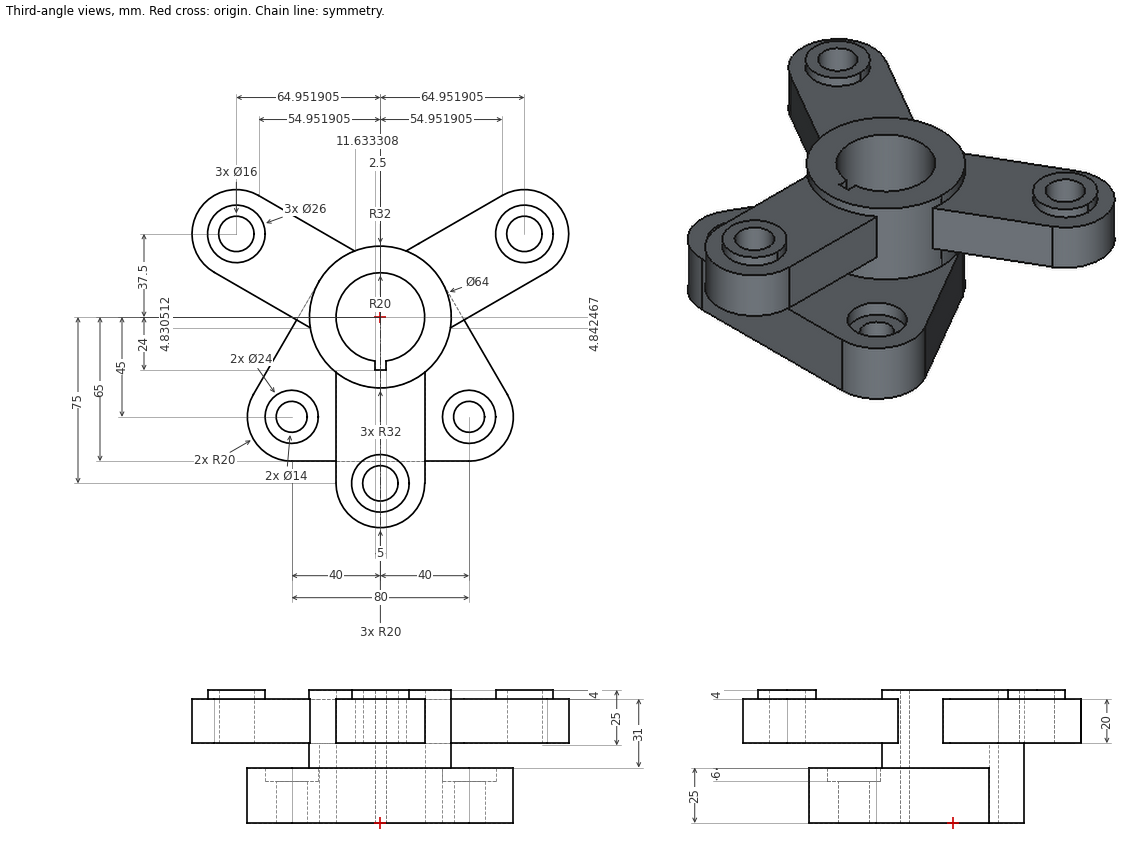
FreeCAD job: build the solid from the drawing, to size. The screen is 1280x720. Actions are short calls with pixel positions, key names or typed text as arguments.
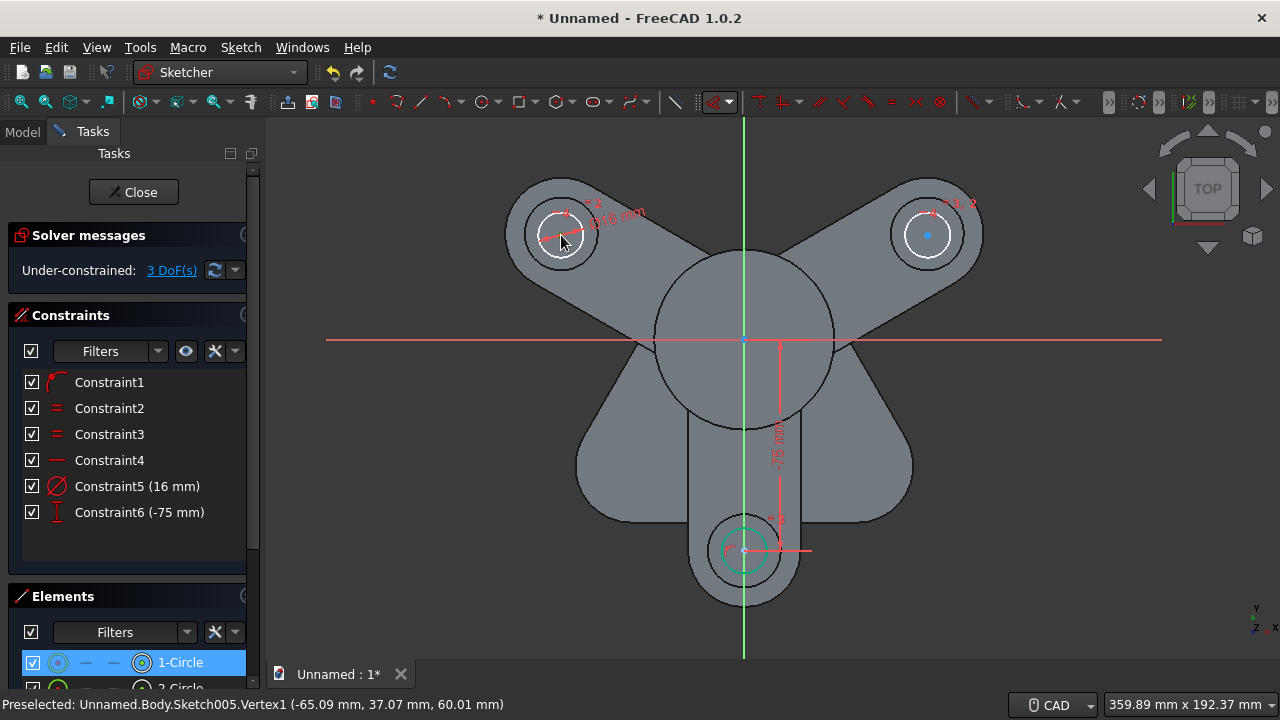
click(732, 102)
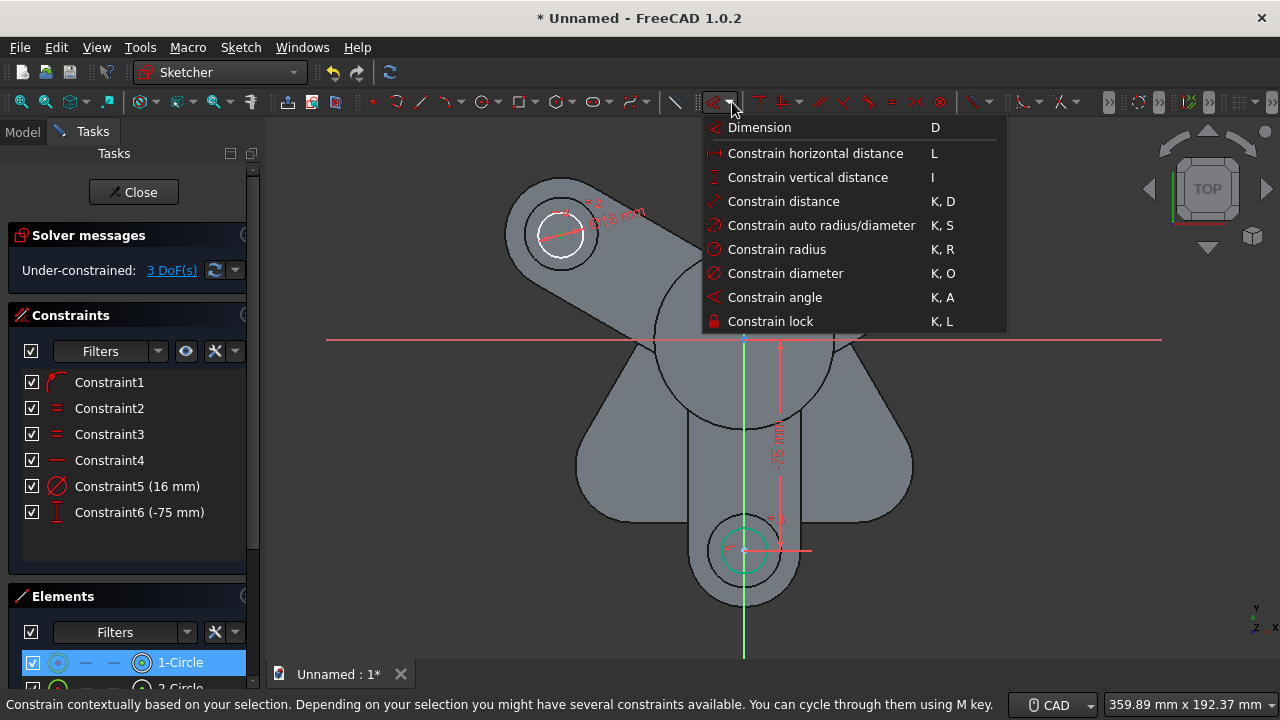
click(855, 177)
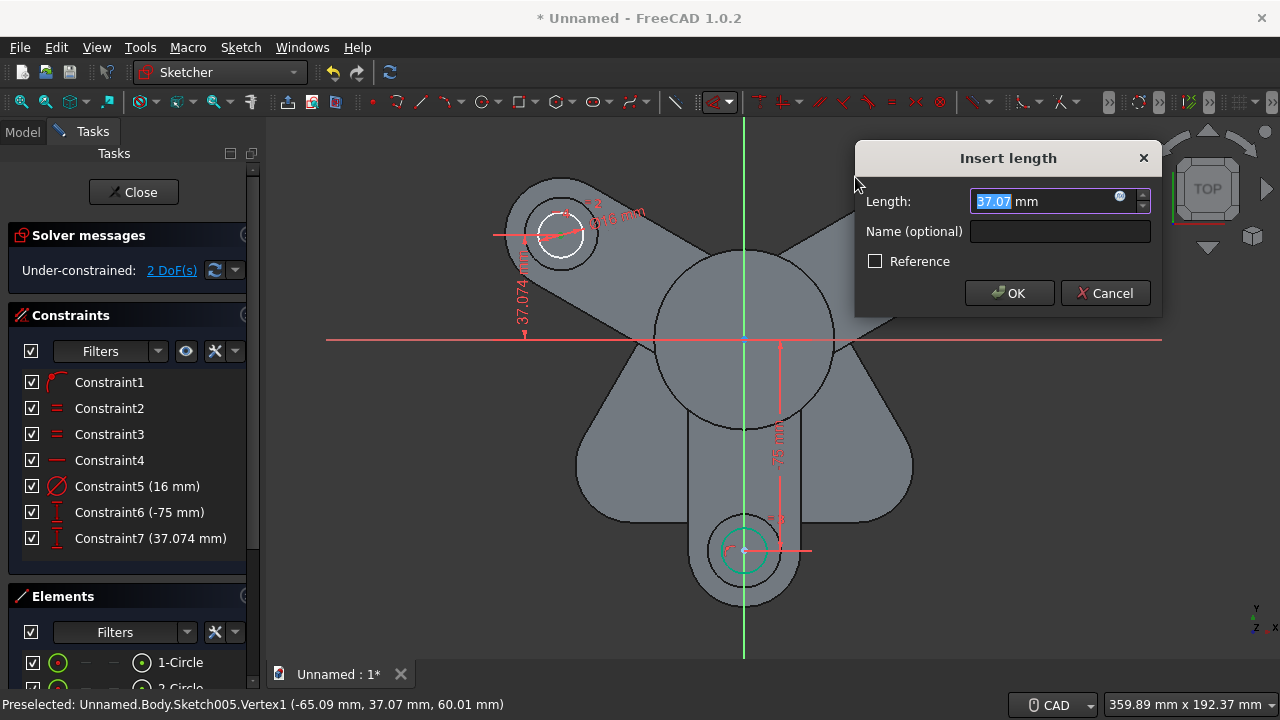
text(37.5)
key(Return)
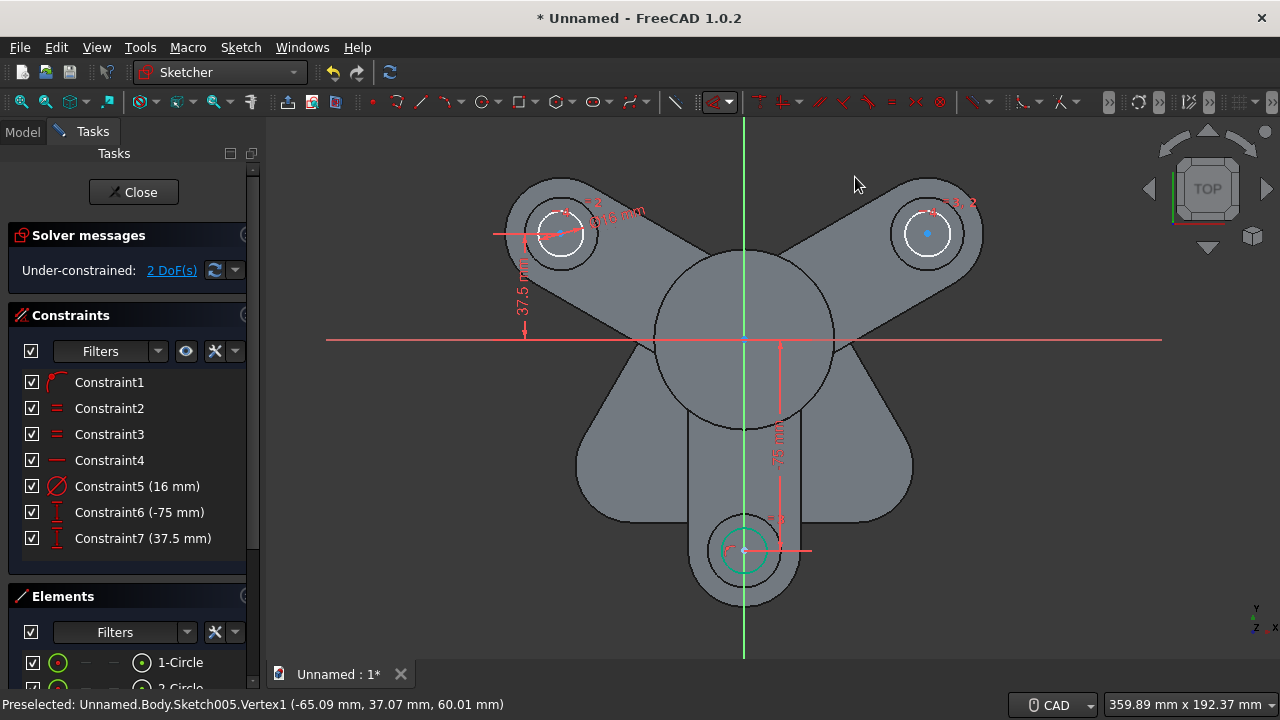
click(561, 234)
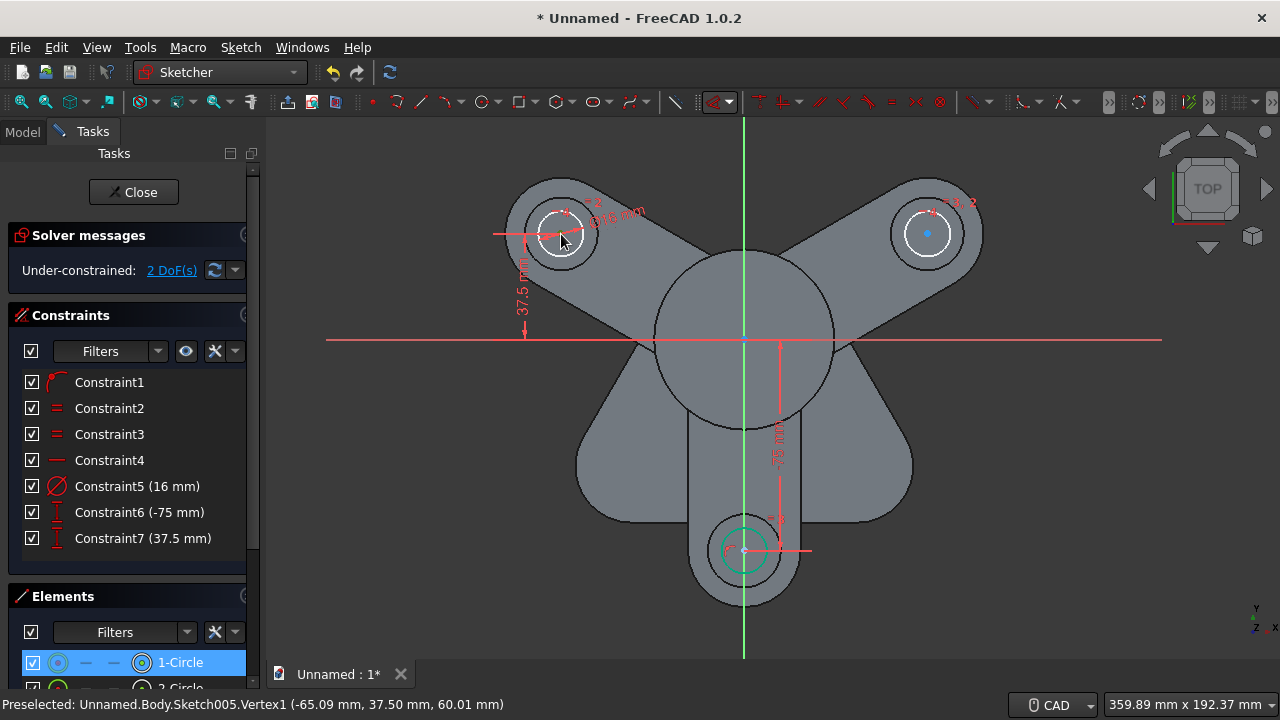
key(l)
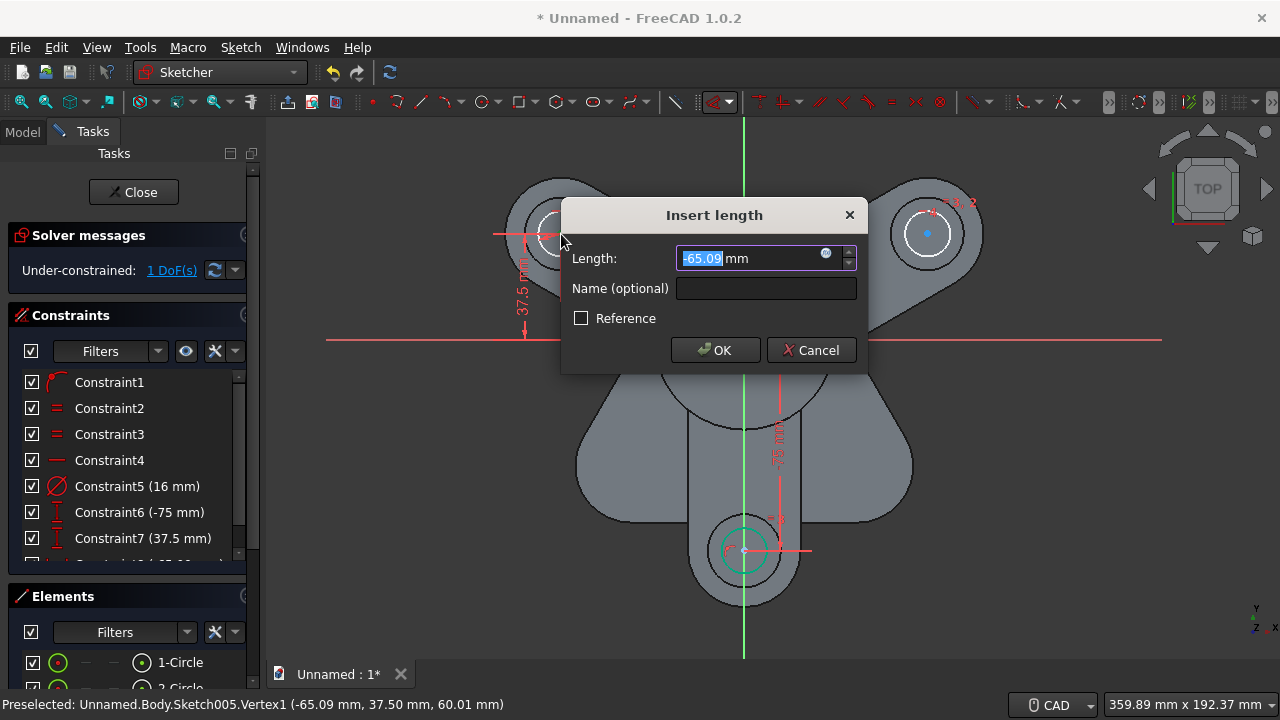
text(-64.951905)
key(Return)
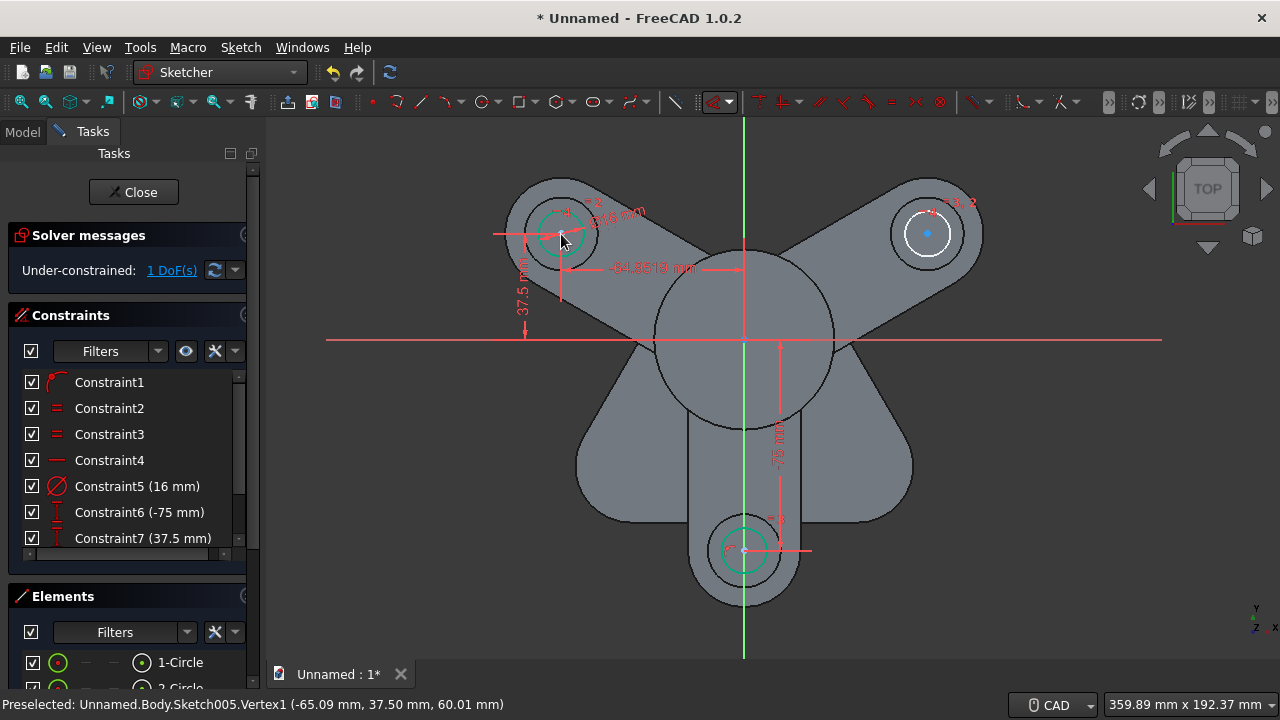
click(928, 234)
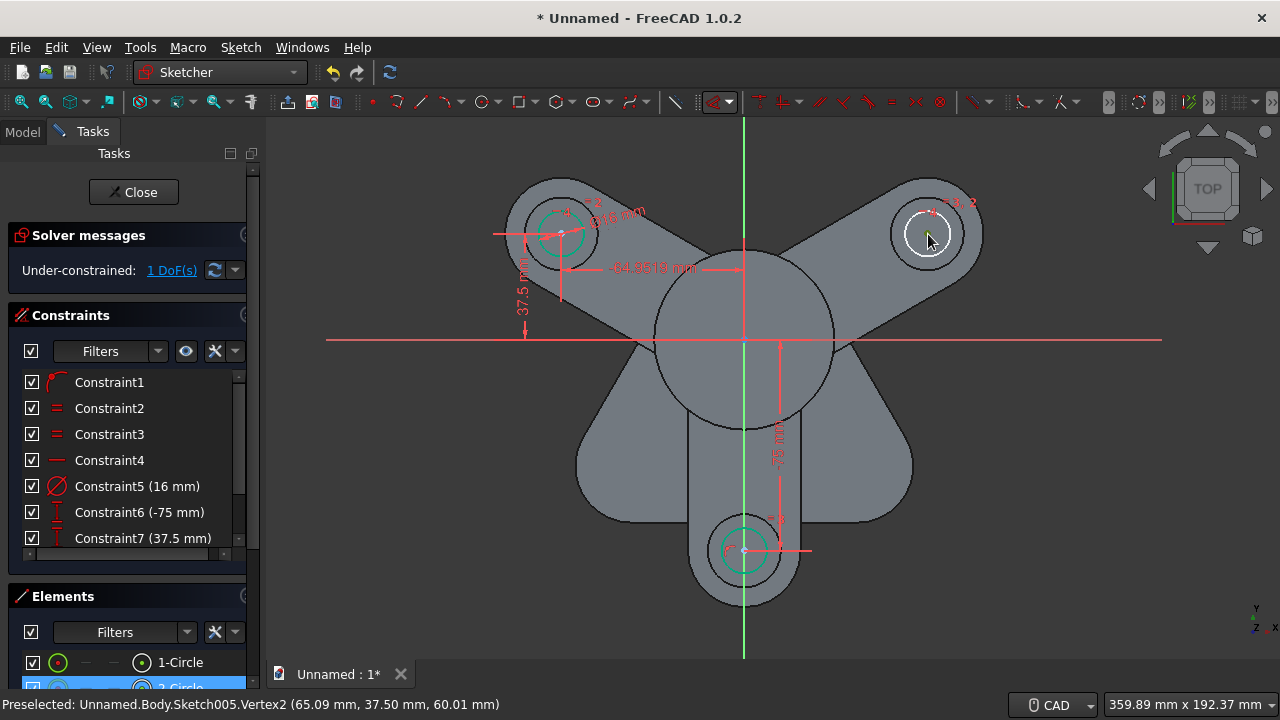
key(l)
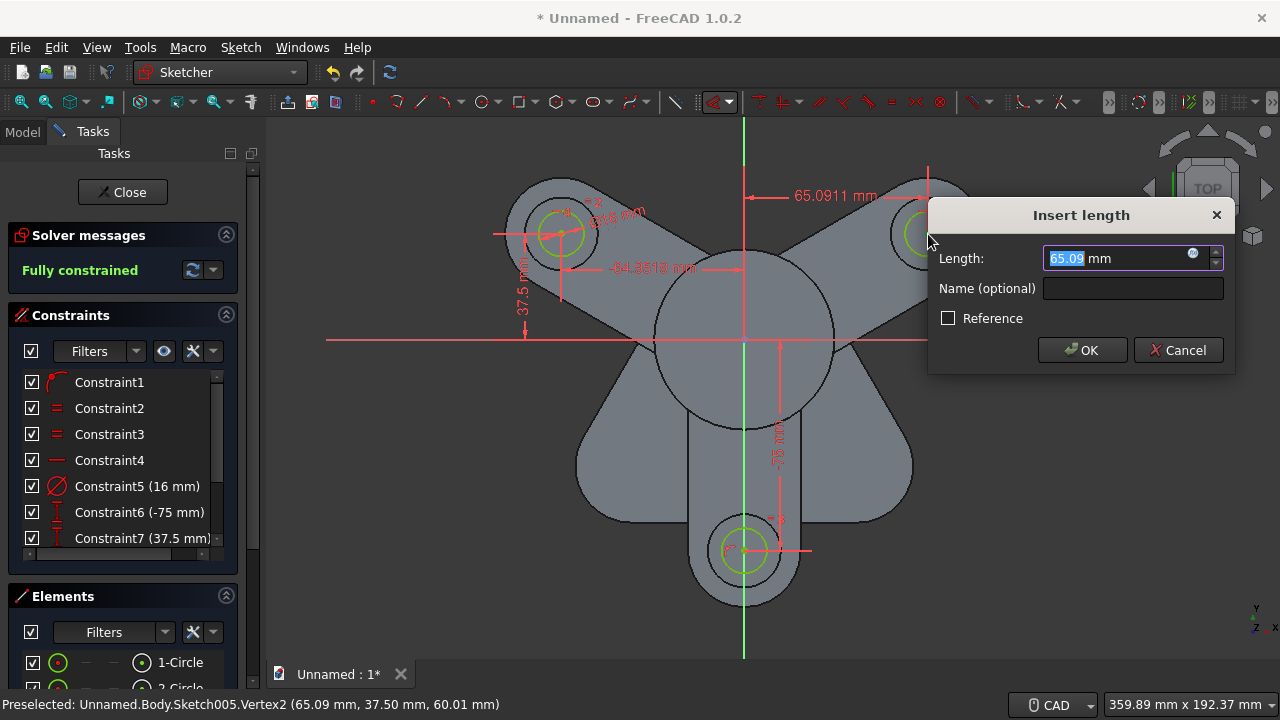
text(64.951905)
key(Return)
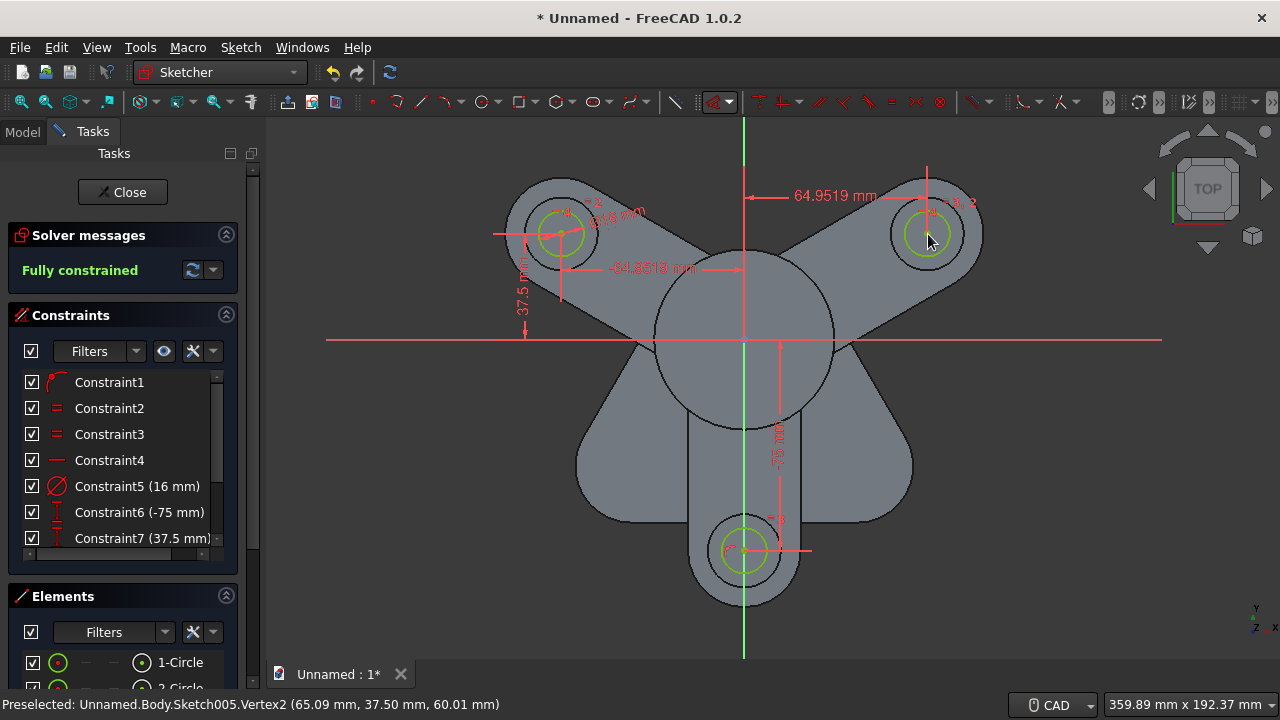
click(123, 192)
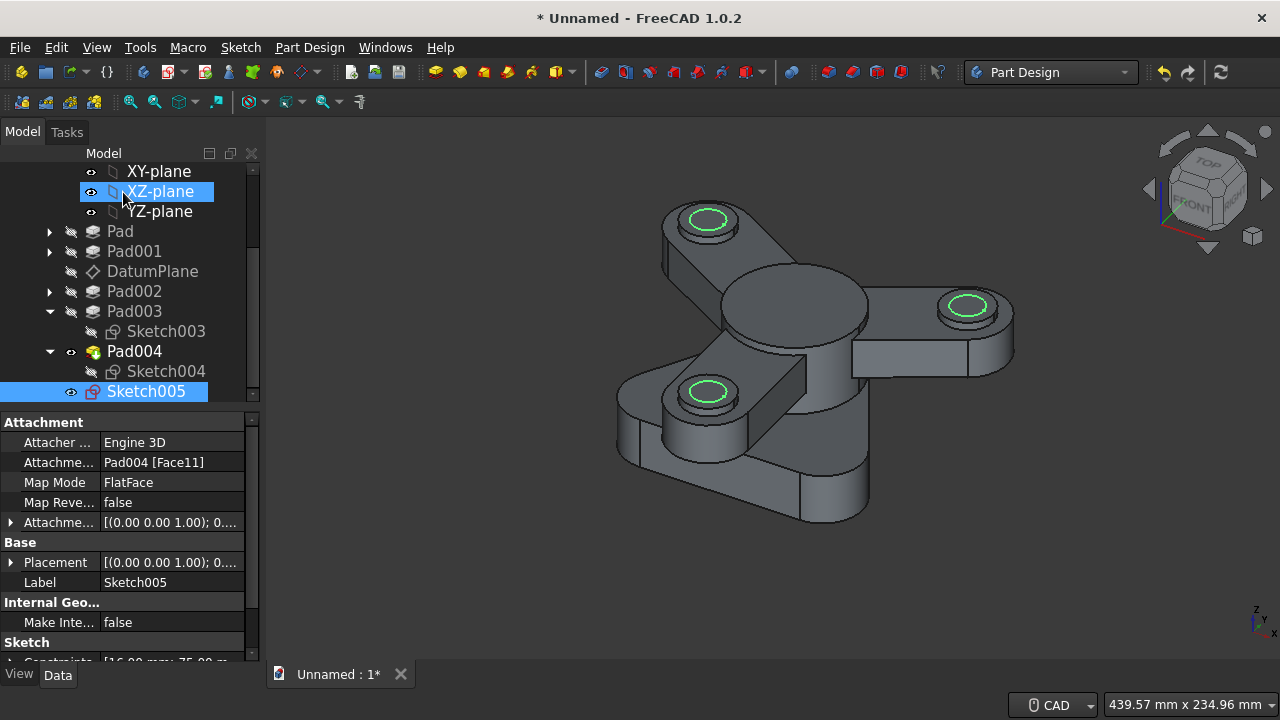
click(602, 72)